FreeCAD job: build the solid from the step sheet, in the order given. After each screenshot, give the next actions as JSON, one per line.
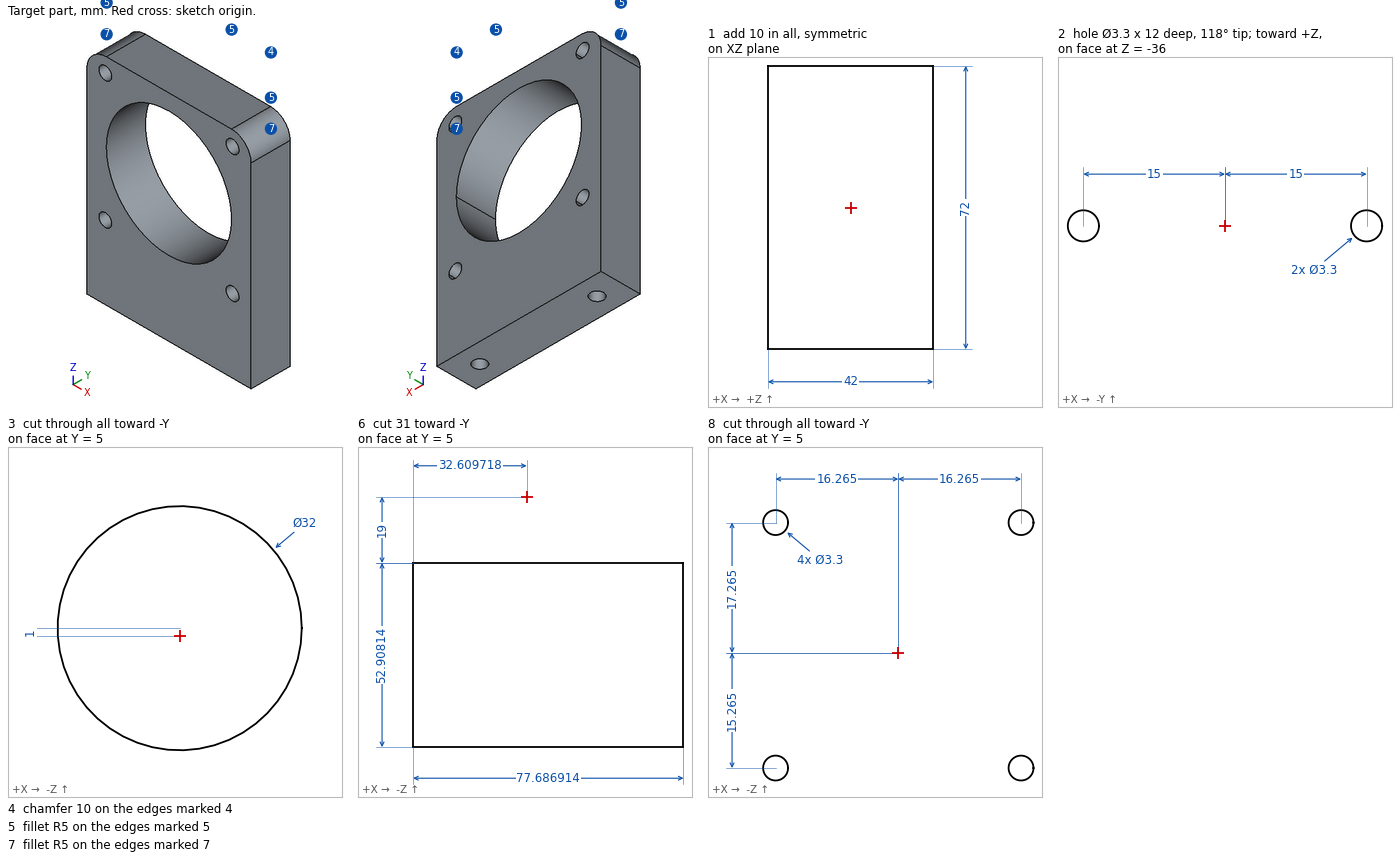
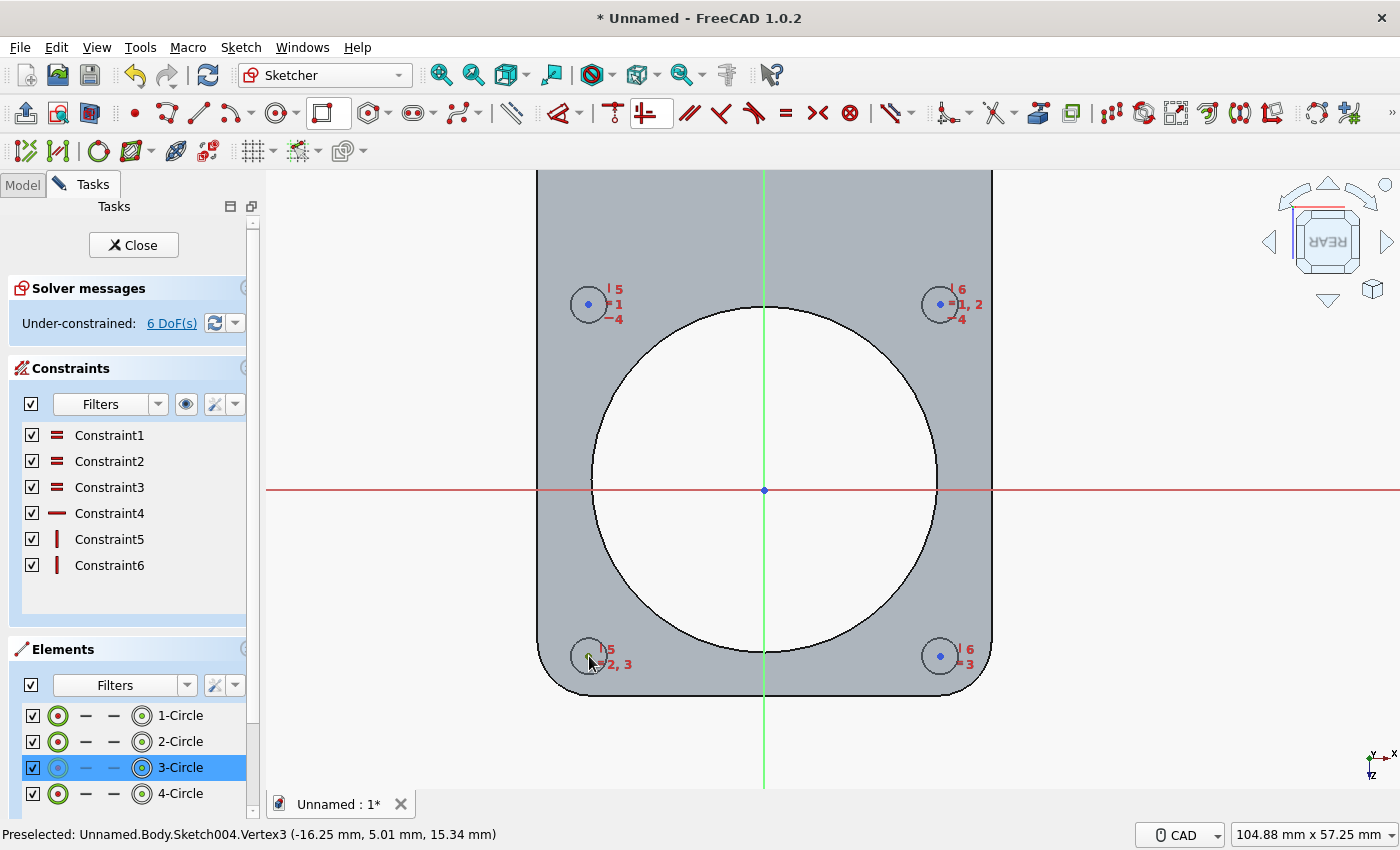
{"action": "left_click", "coordinate": [940, 656]}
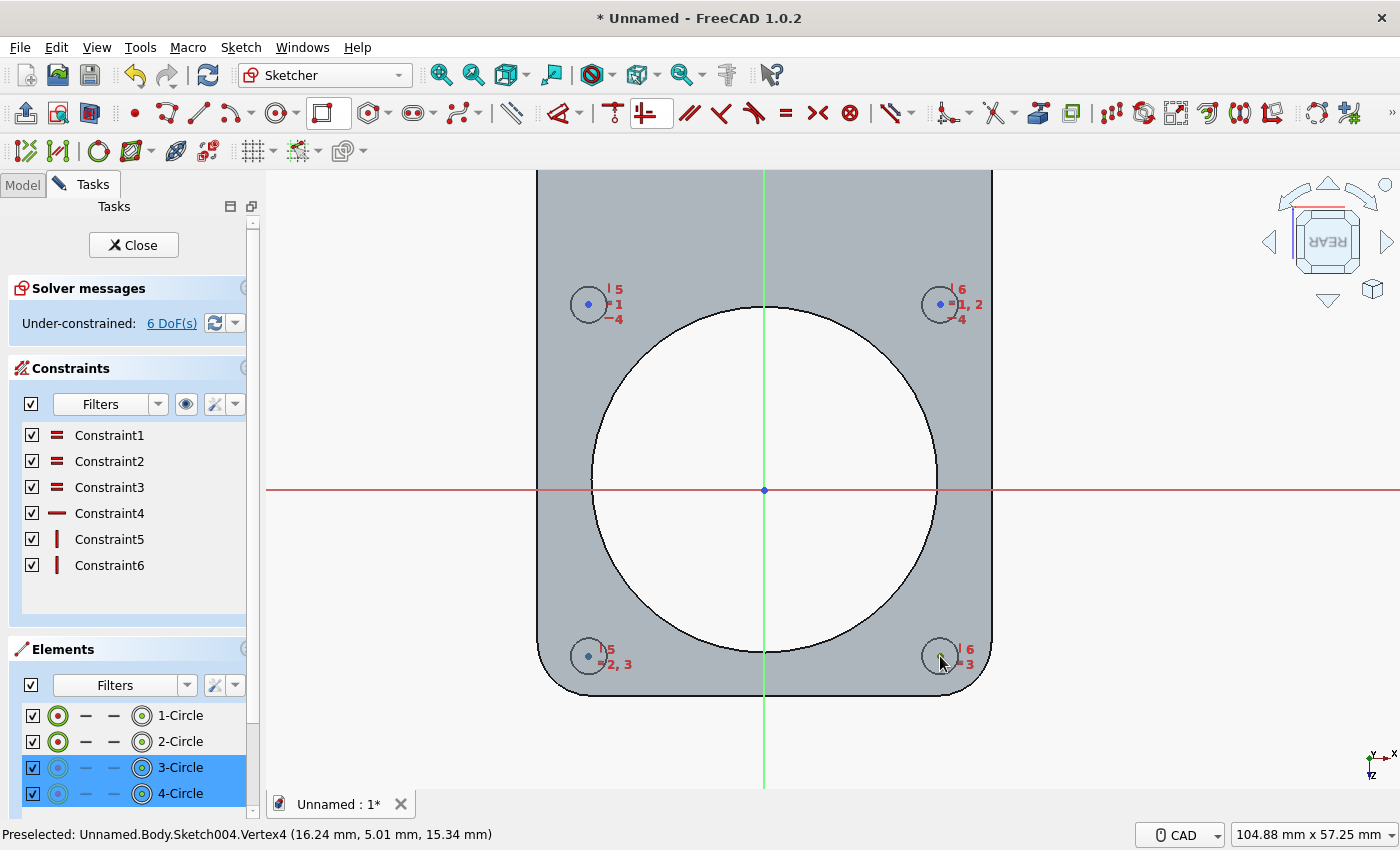
{"action": "key", "text": "h"}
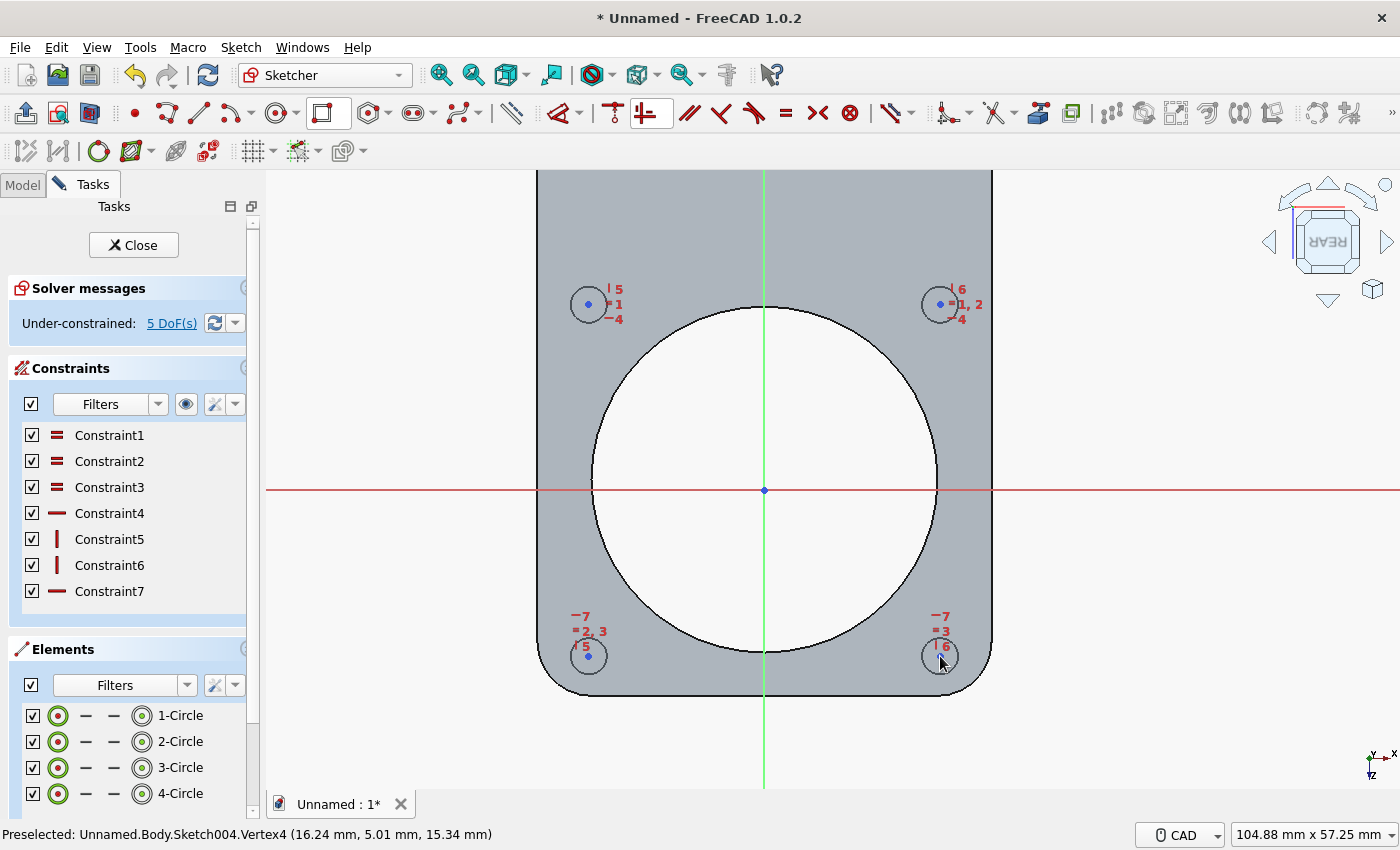
{"action": "left_click", "coordinate": [558, 114]}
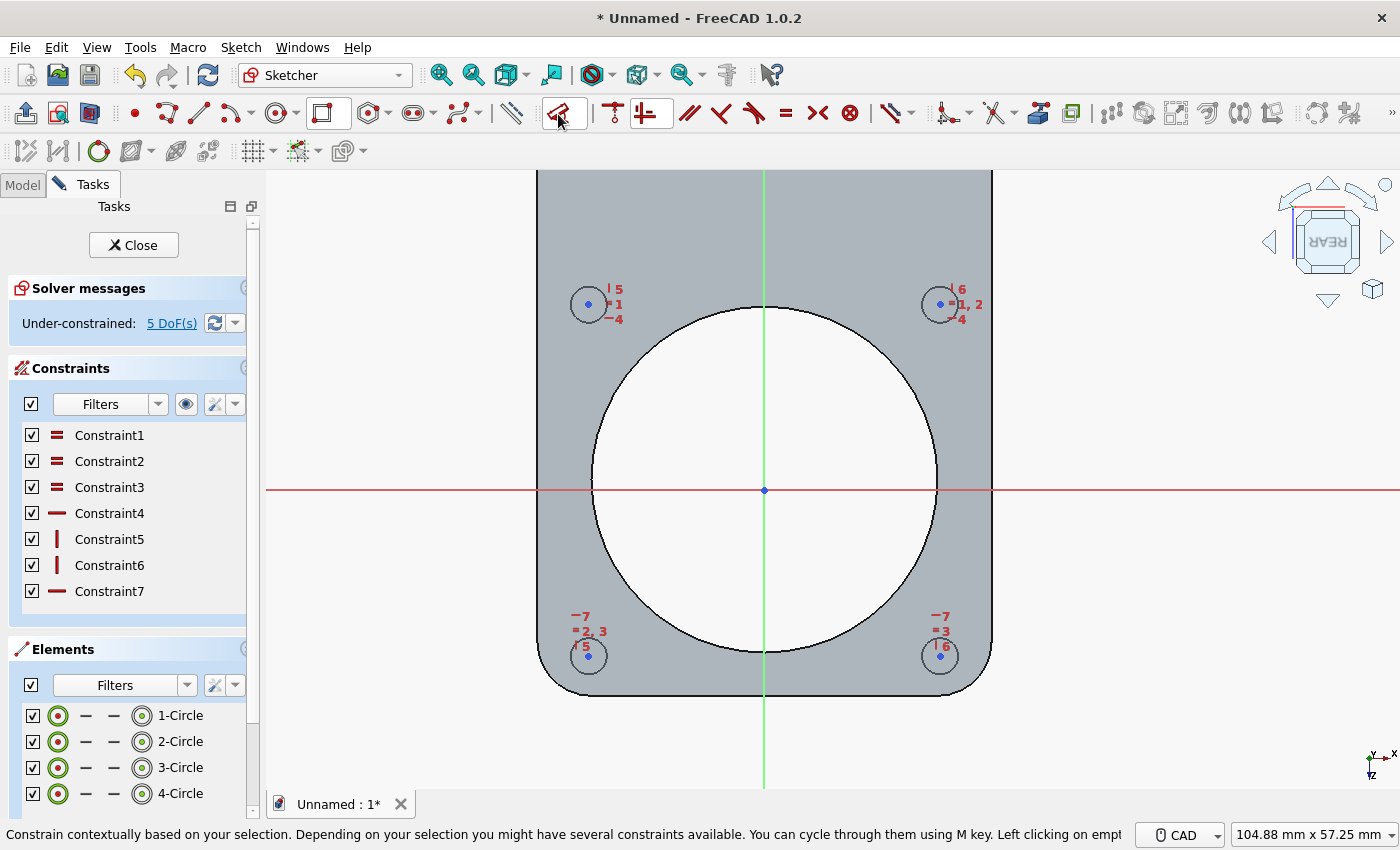
{"action": "left_click", "coordinate": [602, 292]}
{"action": "left_click", "coordinate": [625, 270]}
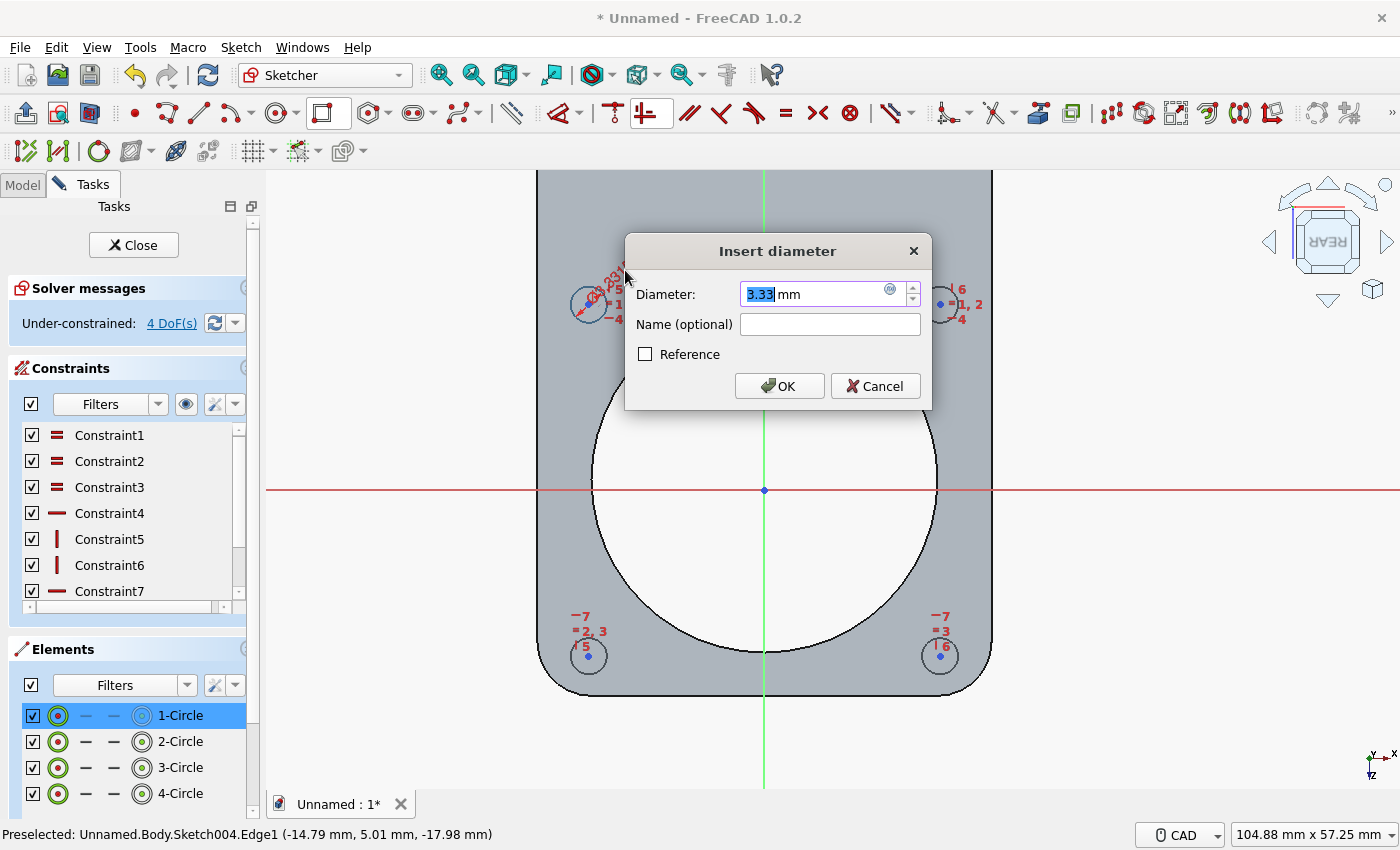
{"action": "type", "text": "3.3"}
{"action": "key", "text": "Return"}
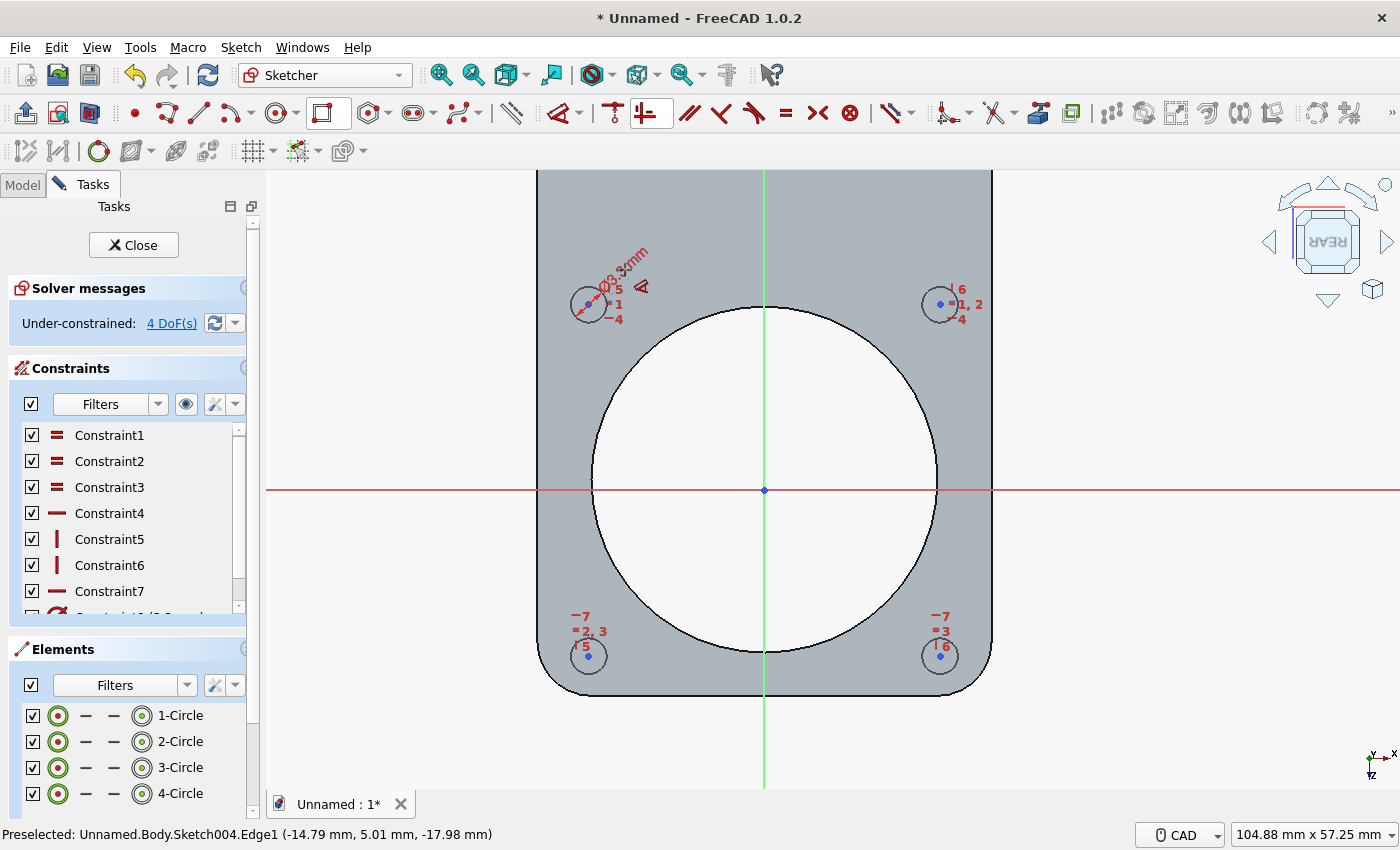
{"action": "left_click", "coordinate": [589, 305]}
{"action": "left_click", "coordinate": [717, 271]}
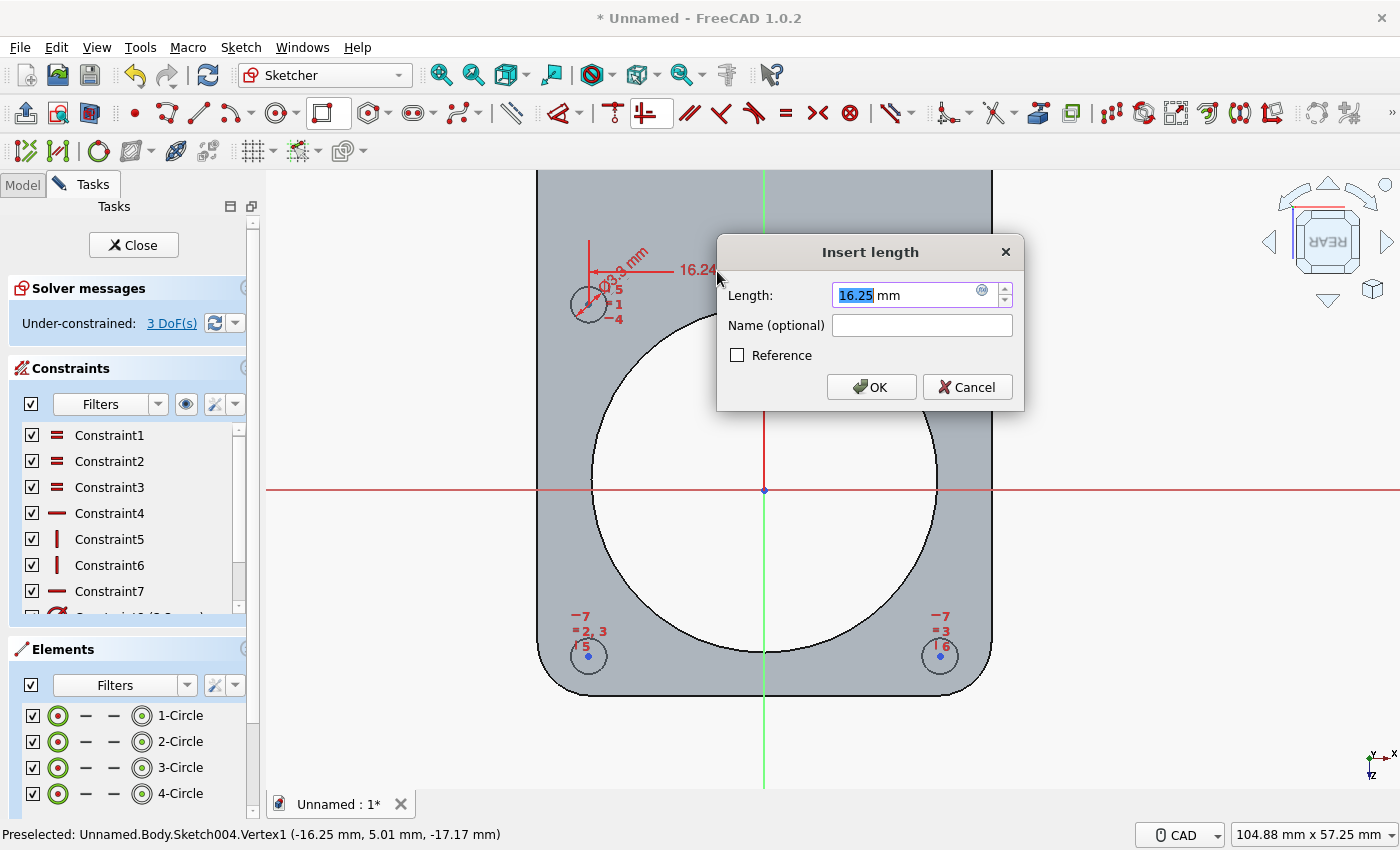
{"action": "type", "text": "16.265"}
{"action": "key", "text": "Return"}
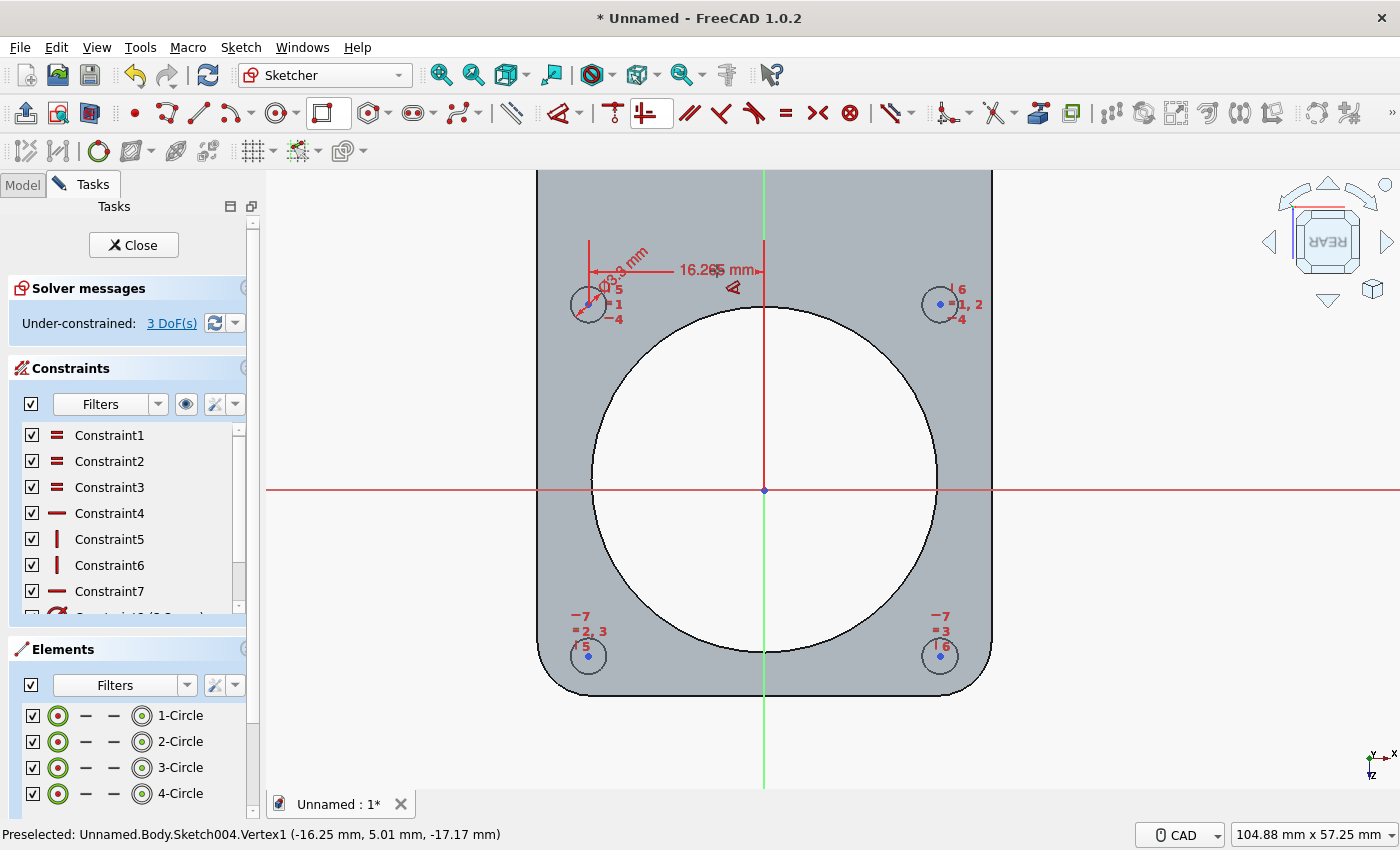
{"action": "left_click", "coordinate": [589, 305]}
{"action": "left_click", "coordinate": [555, 398]}